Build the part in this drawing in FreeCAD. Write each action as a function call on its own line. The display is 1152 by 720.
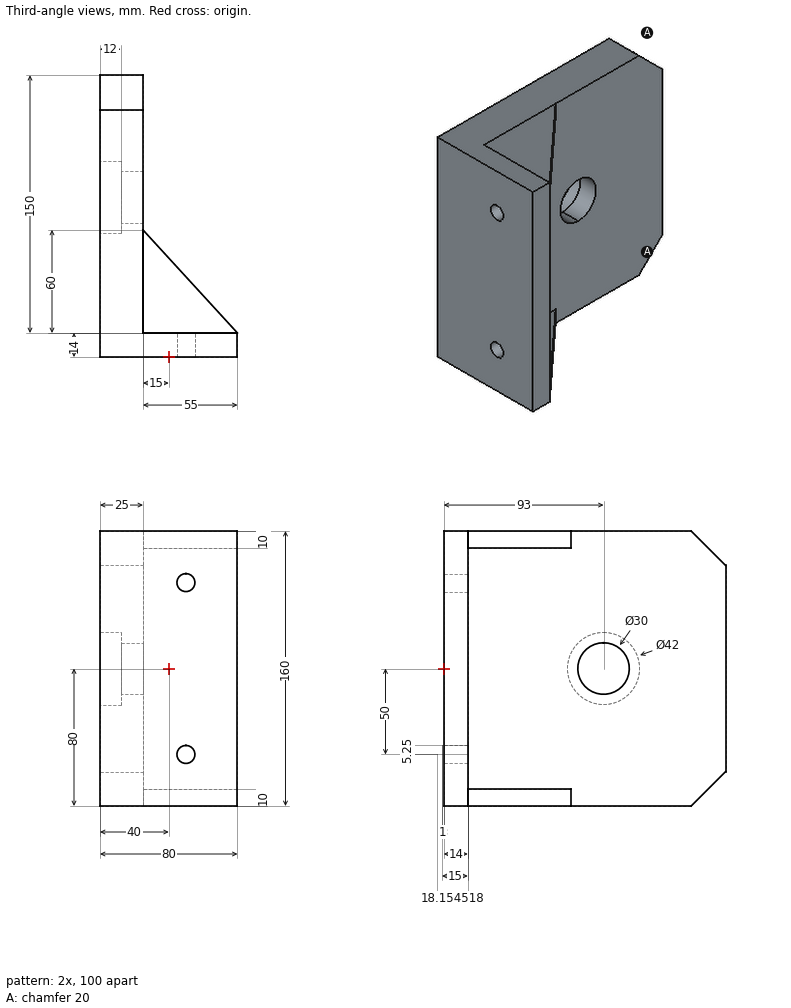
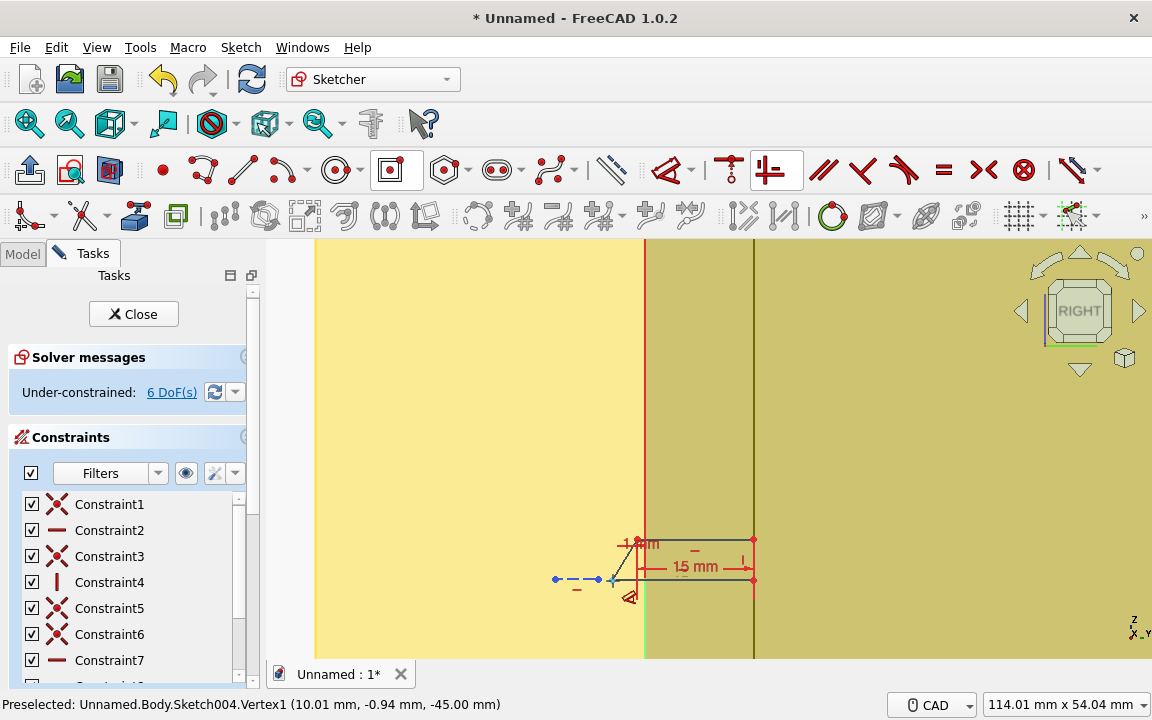
click(612, 580)
click(578, 424)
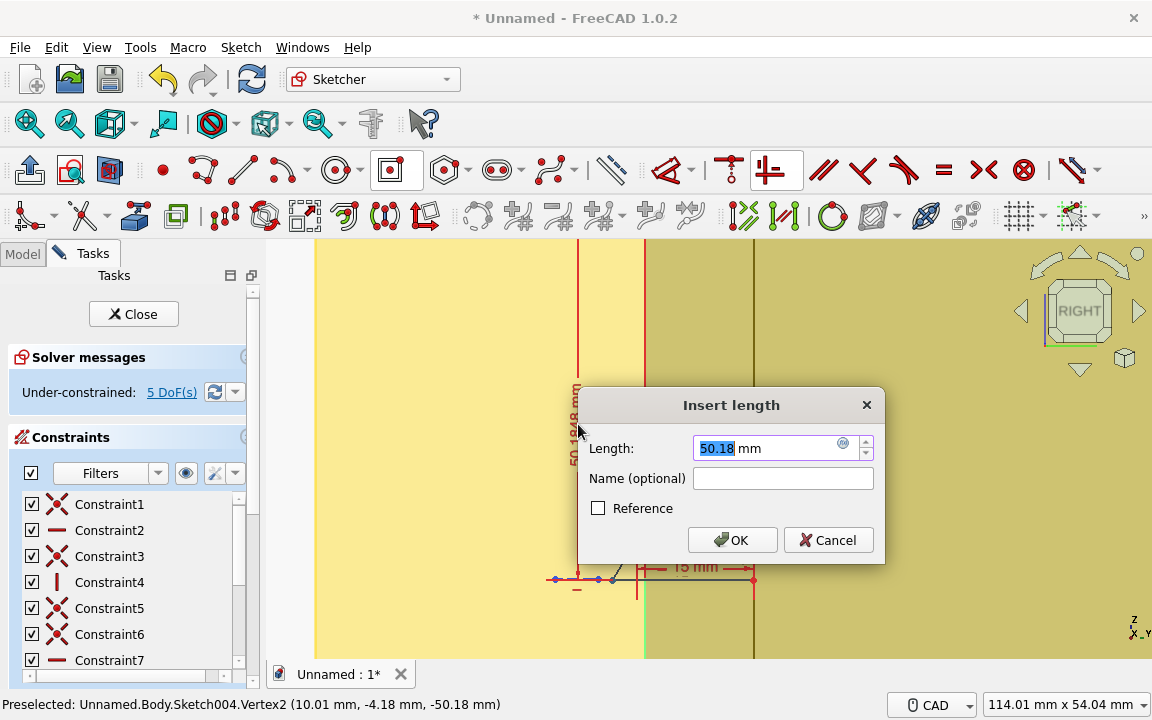
text(50)
key(Return)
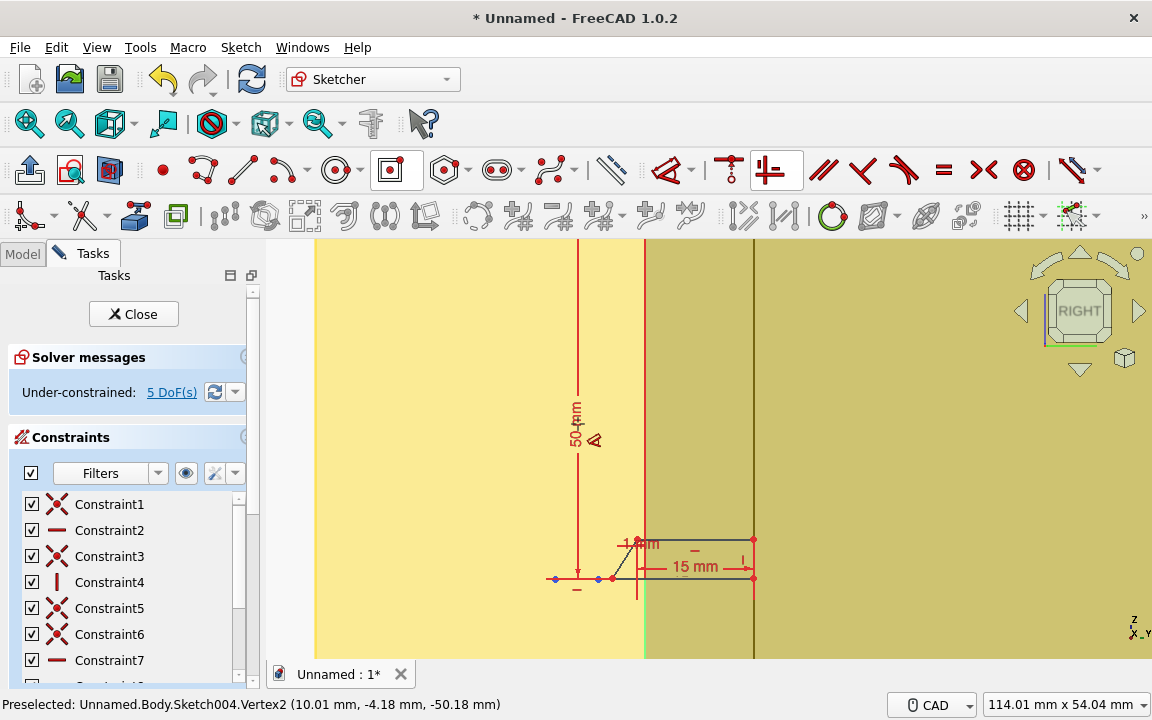
click(598, 579)
click(564, 351)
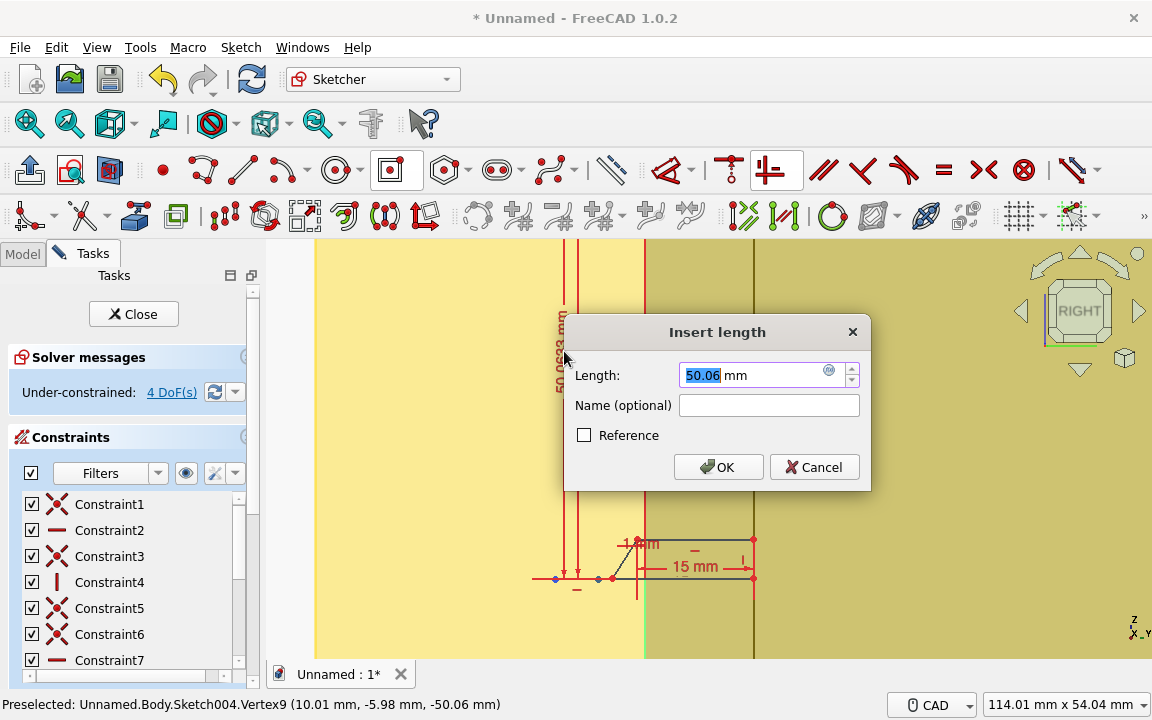
text(50)
key(Return)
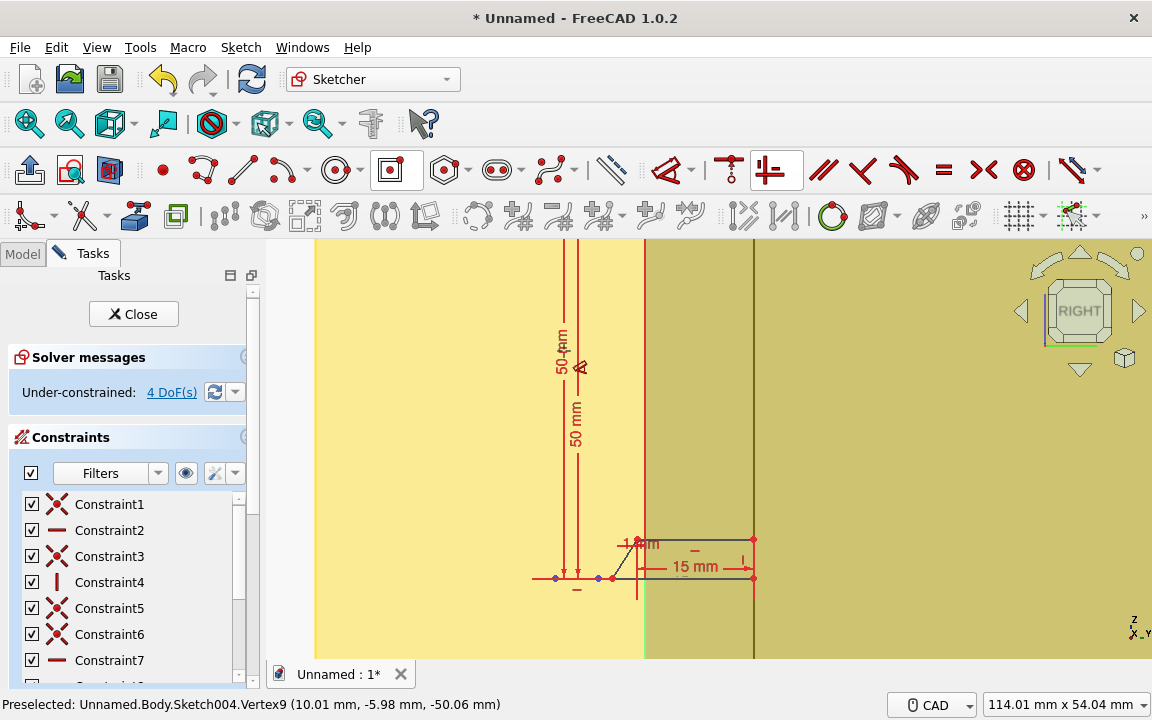
click(754, 567)
click(788, 559)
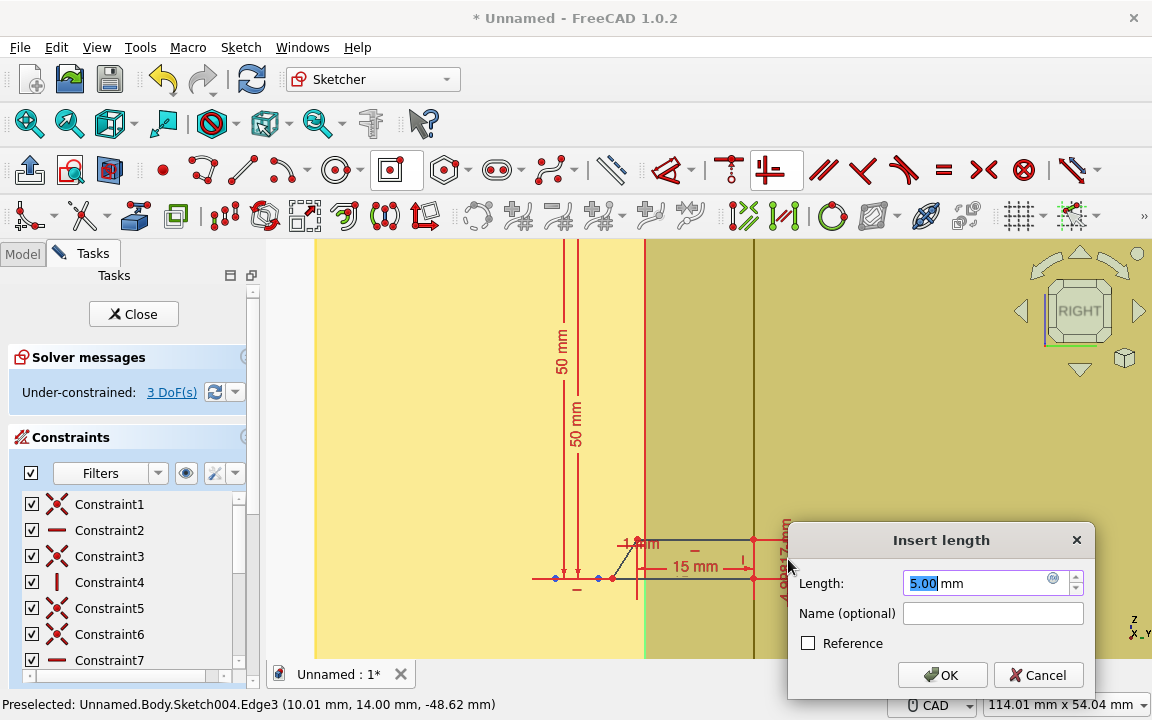
text(5.25)
key(Return)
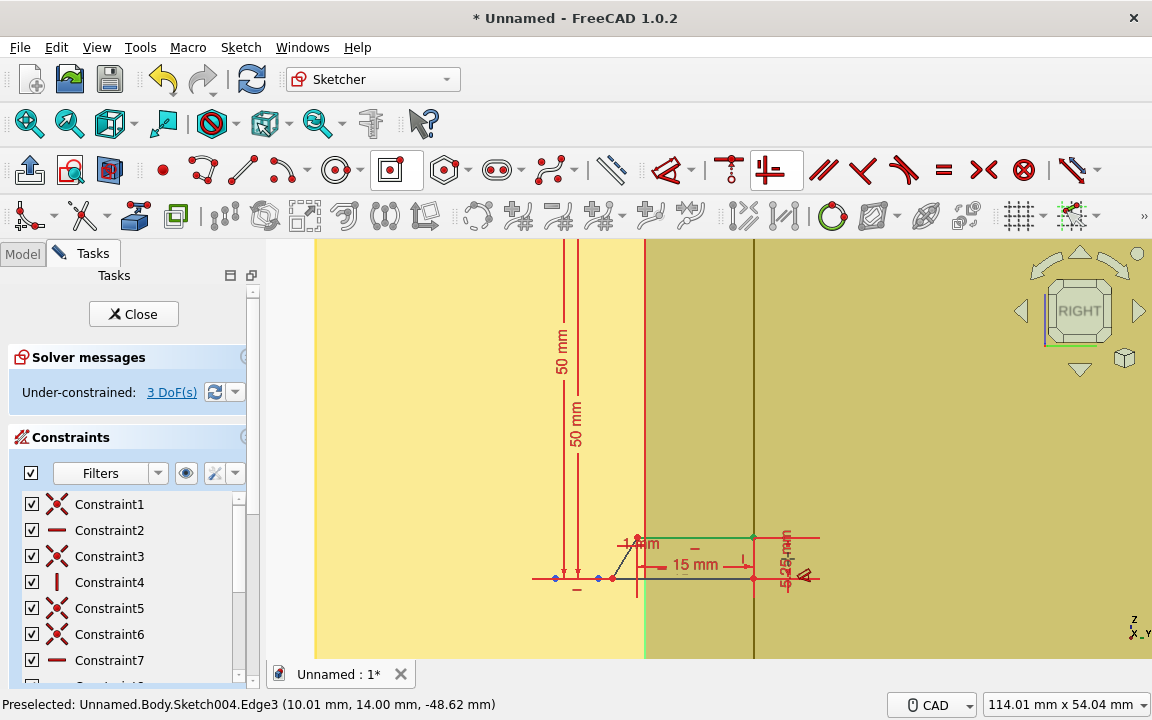
scroll(655, 579, up, 2)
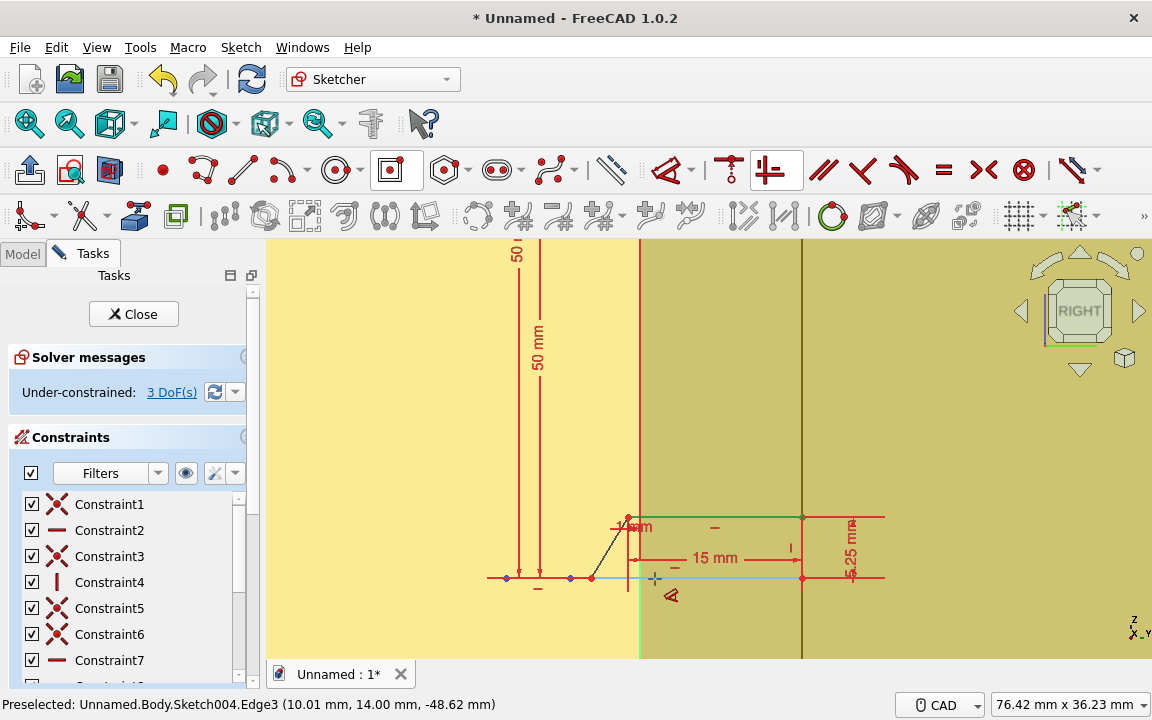
click(655, 578)
click(697, 612)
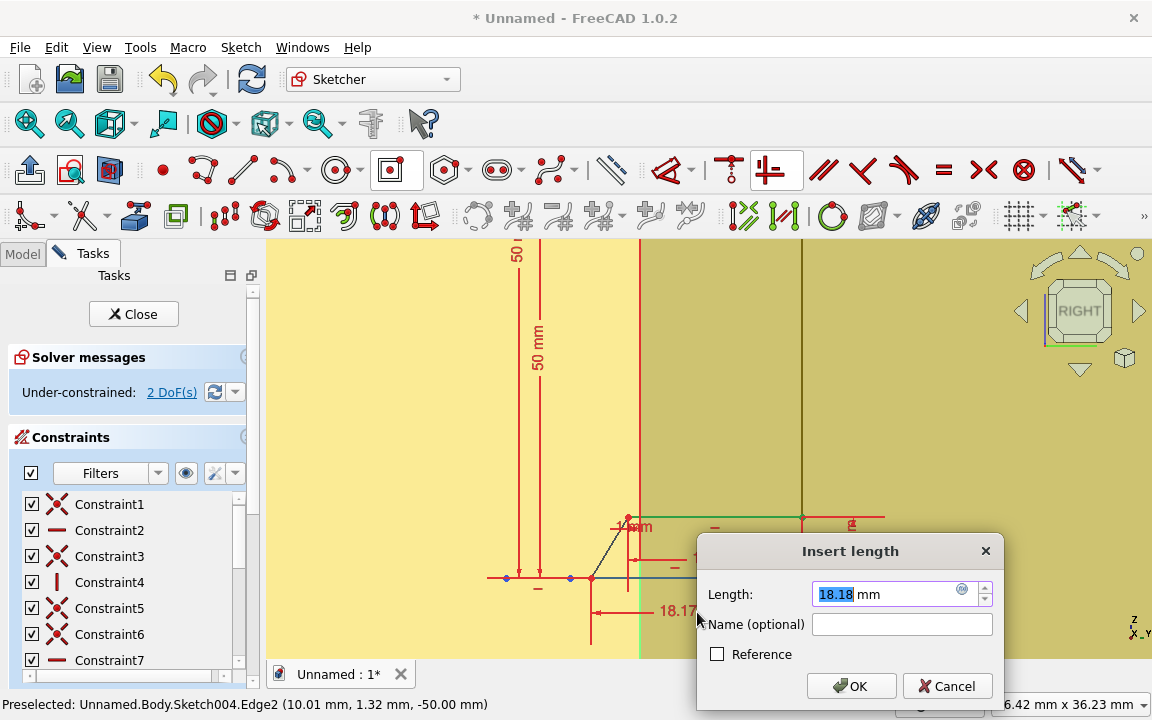
text(18.154518)
key(Return)
key(Escape)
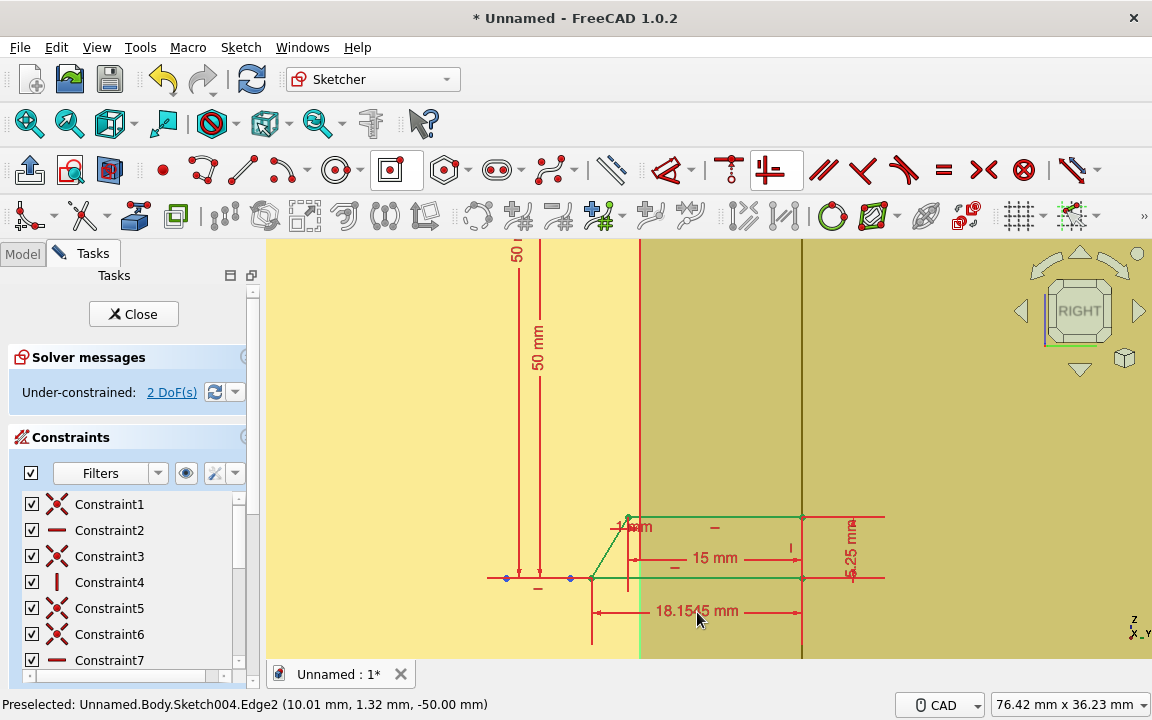
click(134, 314)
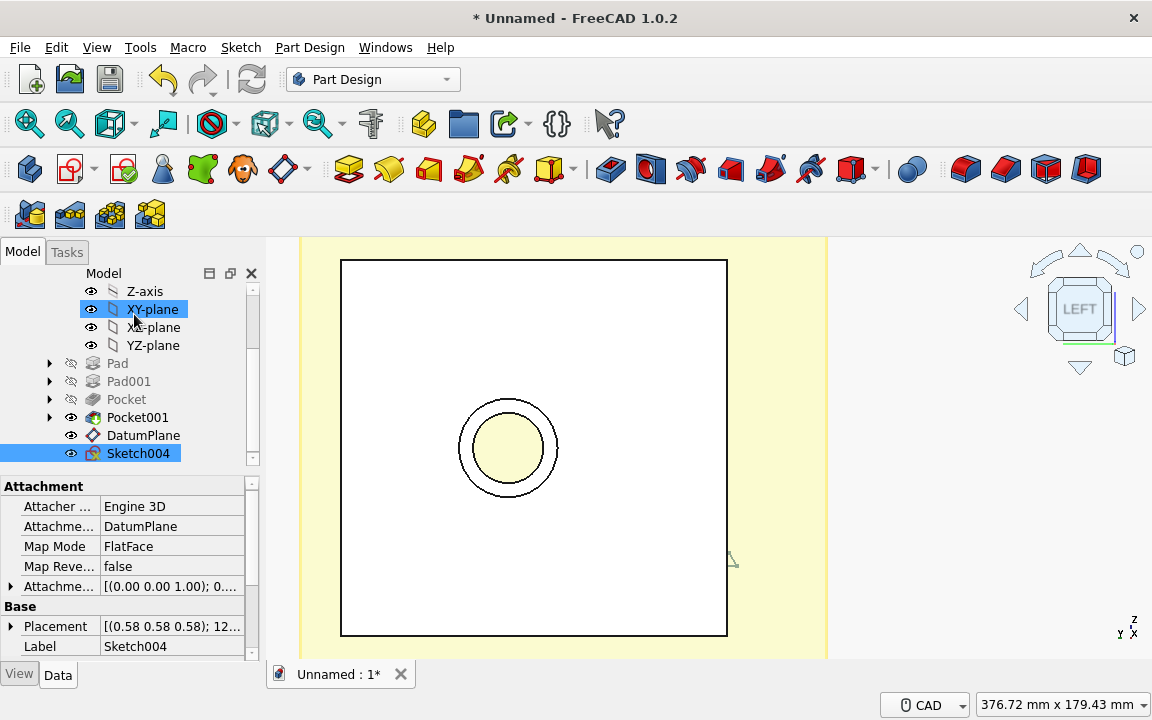
click(692, 170)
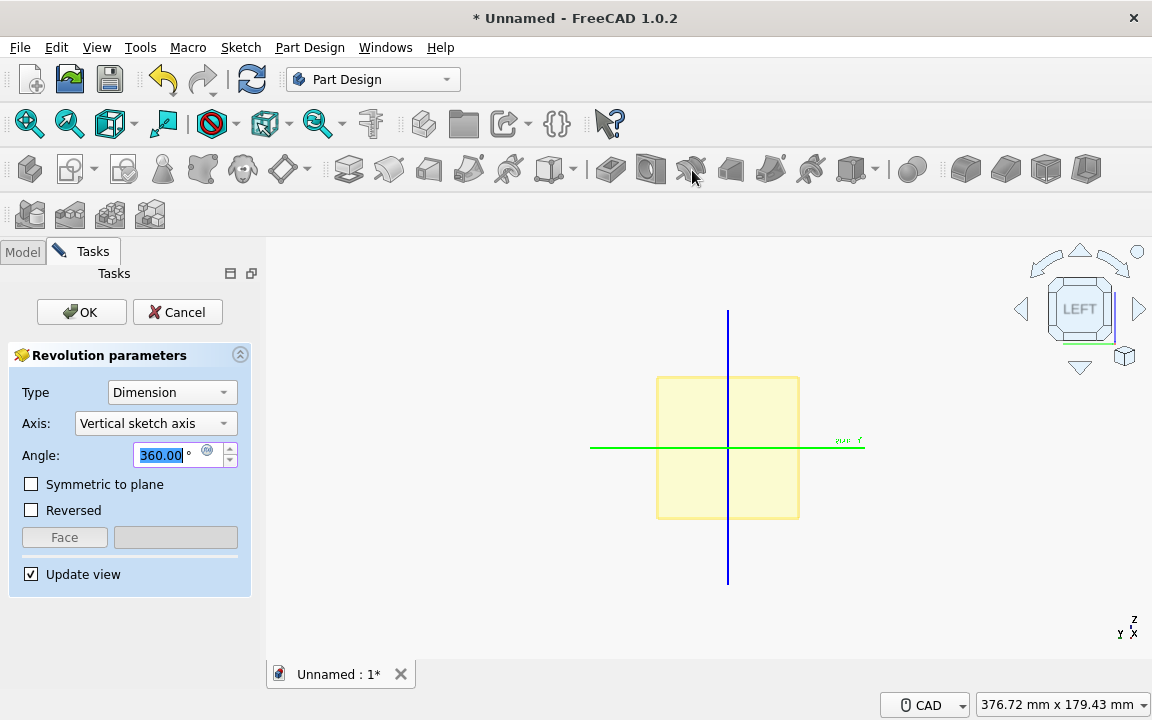
click(156, 424)